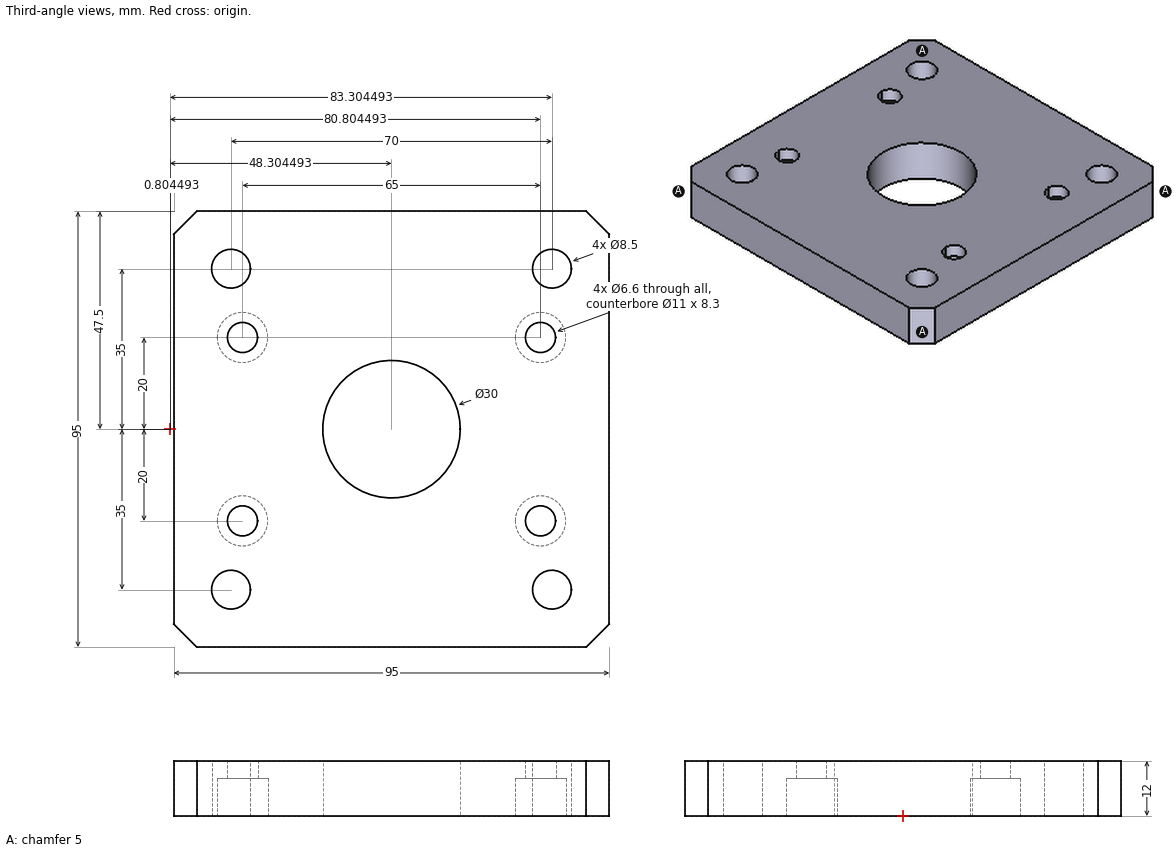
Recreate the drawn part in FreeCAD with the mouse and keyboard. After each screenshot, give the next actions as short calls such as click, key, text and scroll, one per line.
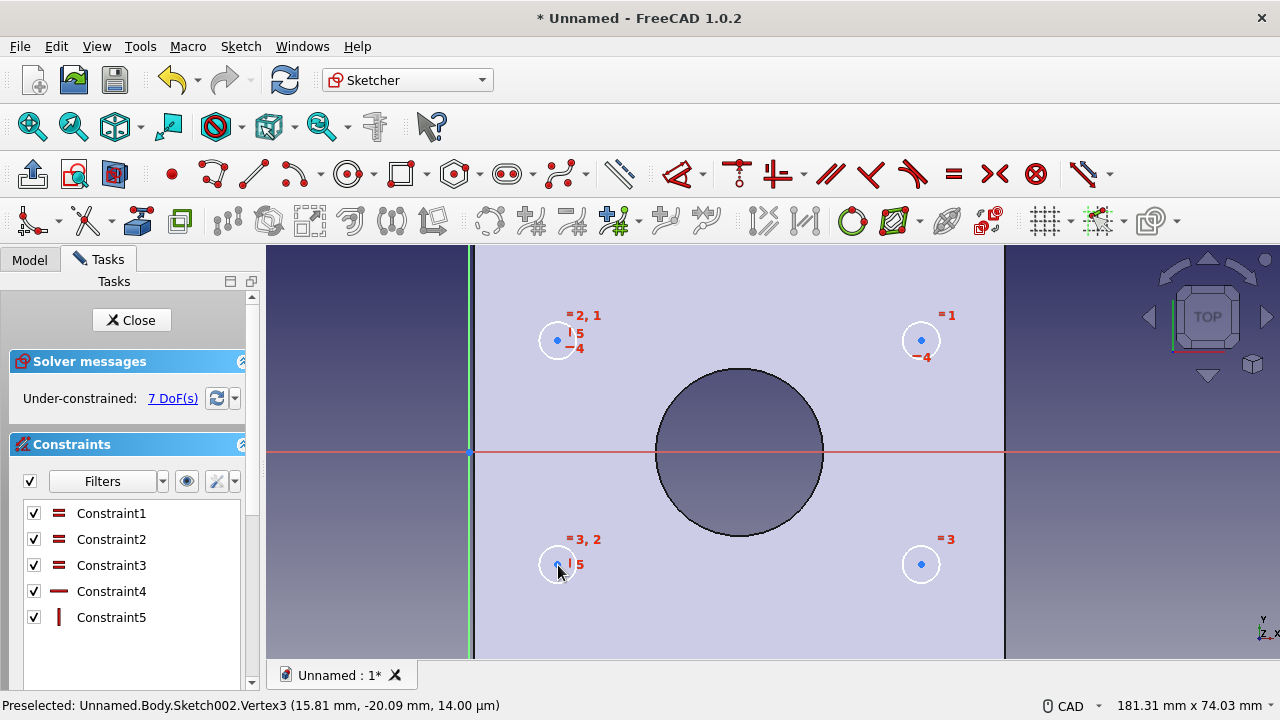
click(921, 341)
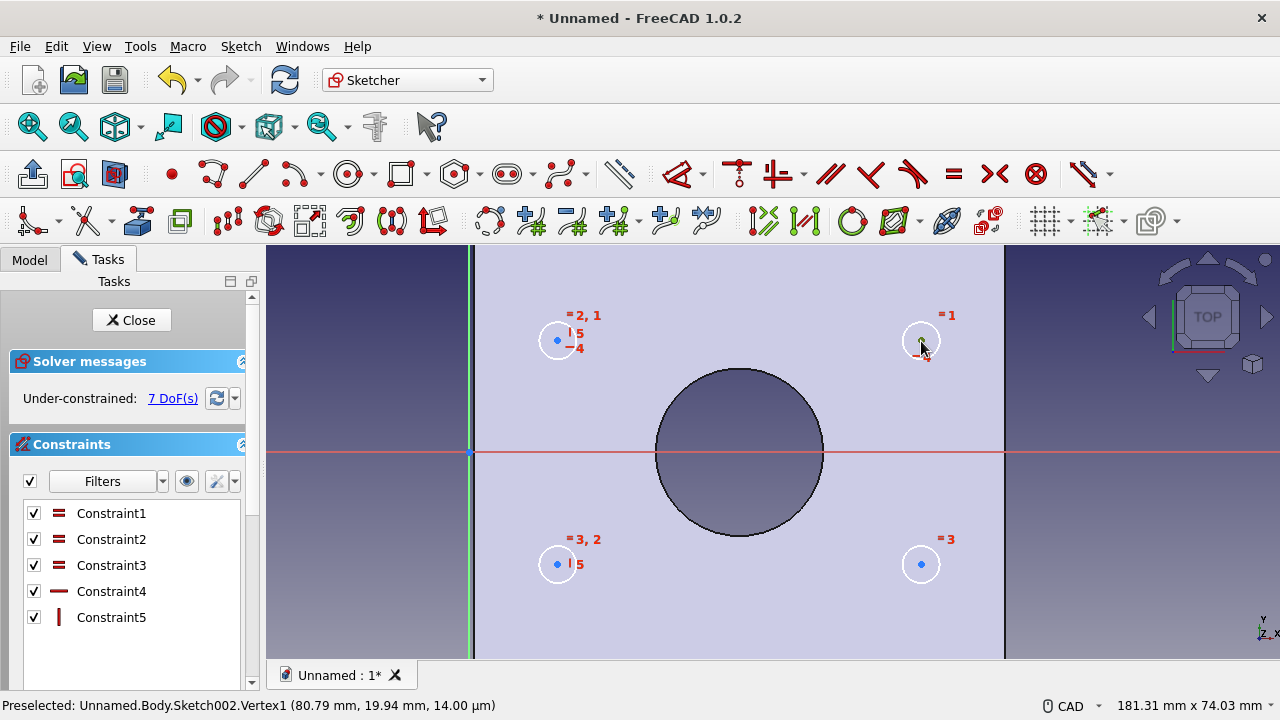
click(921, 565)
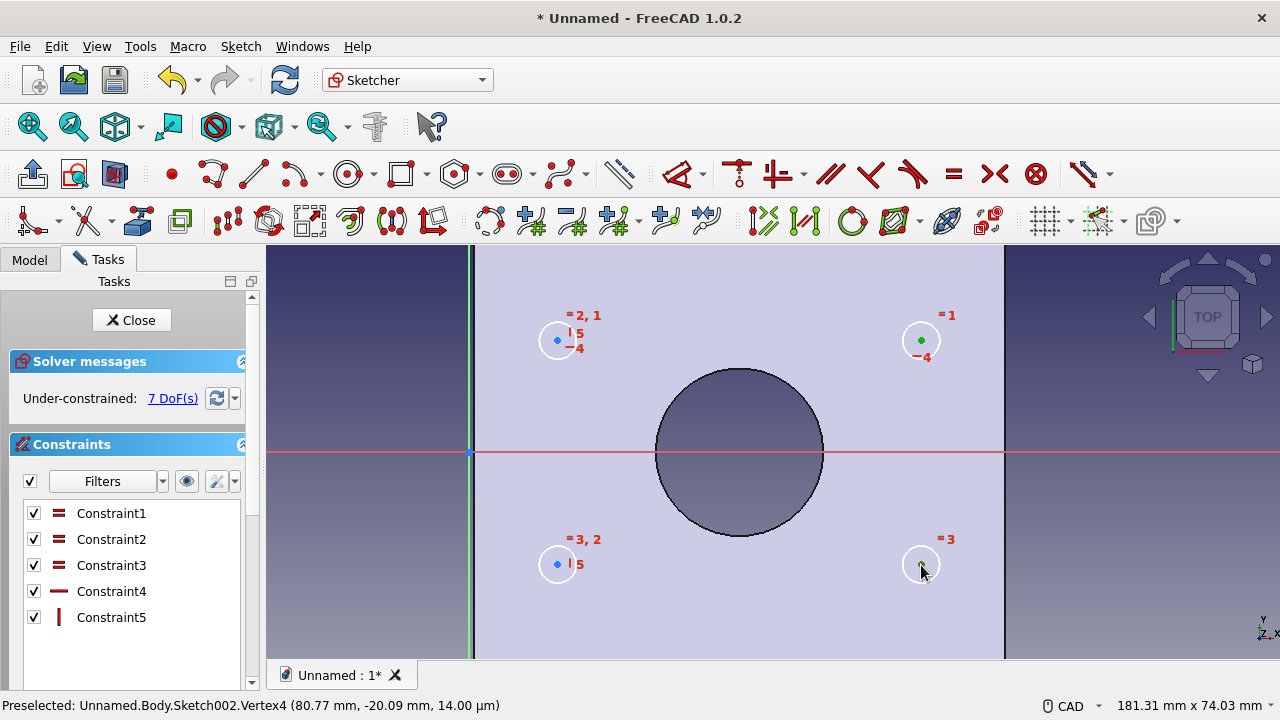
key(v)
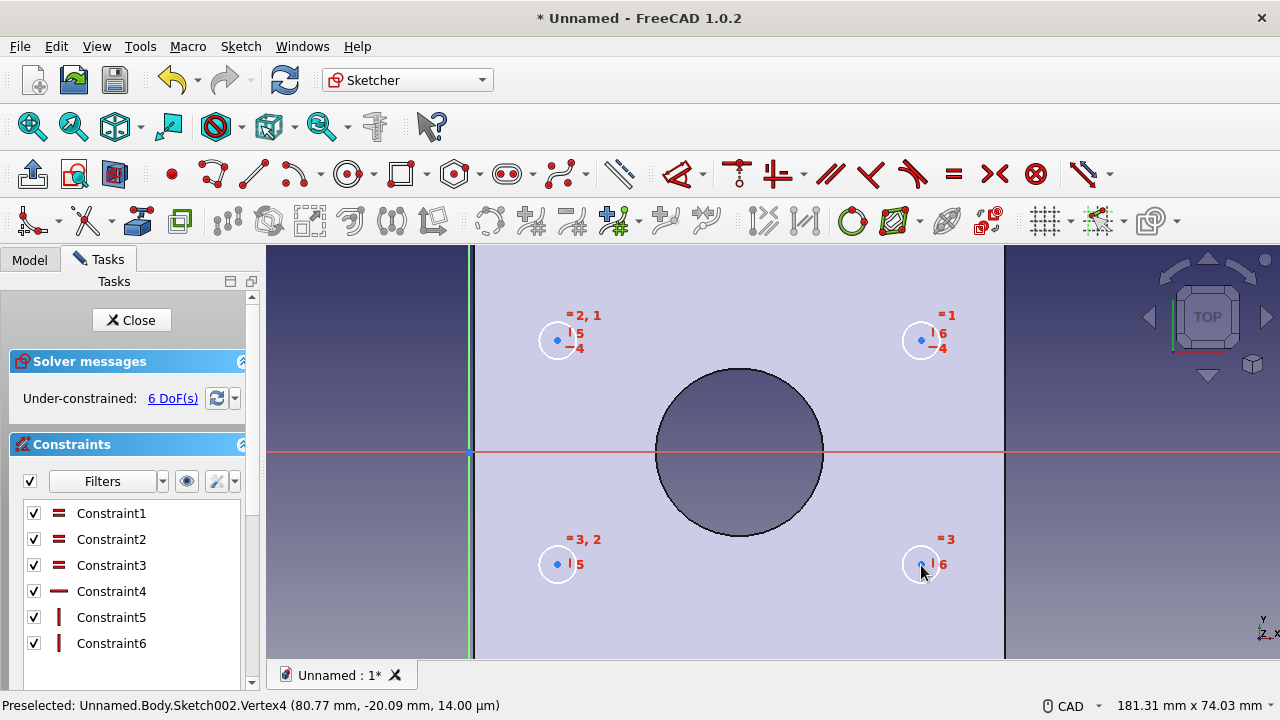
click(558, 565)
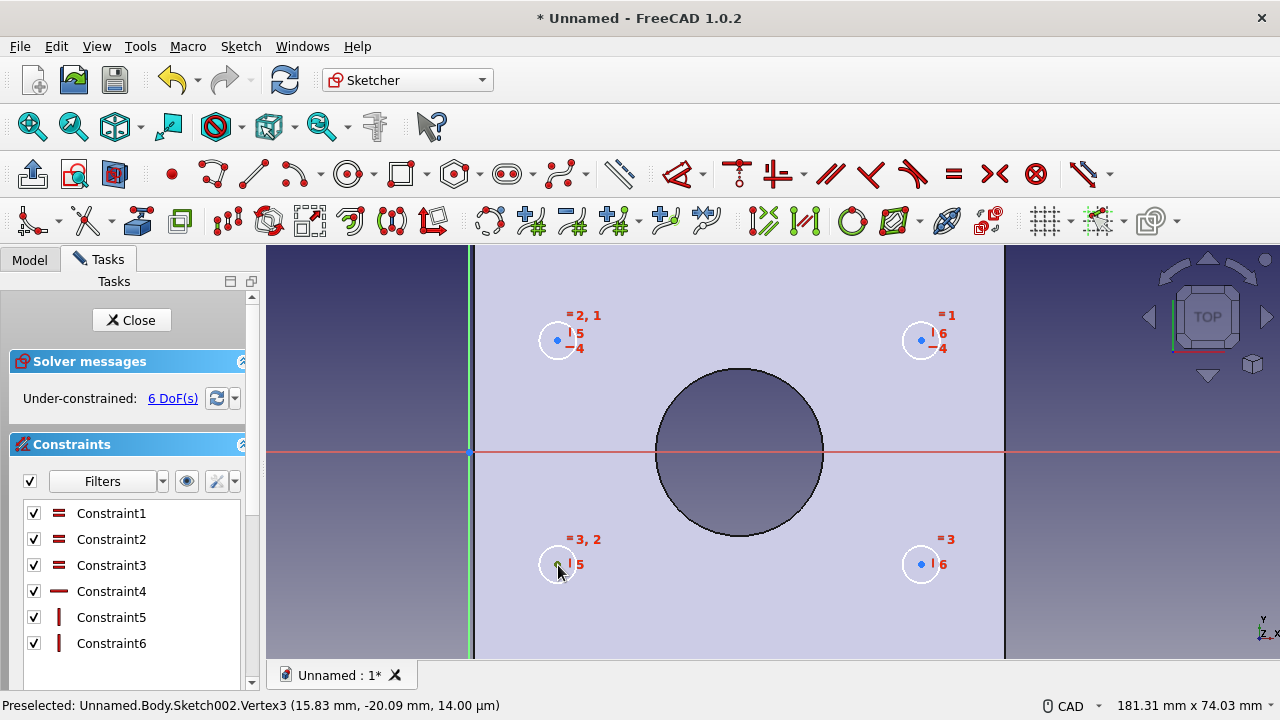
click(921, 565)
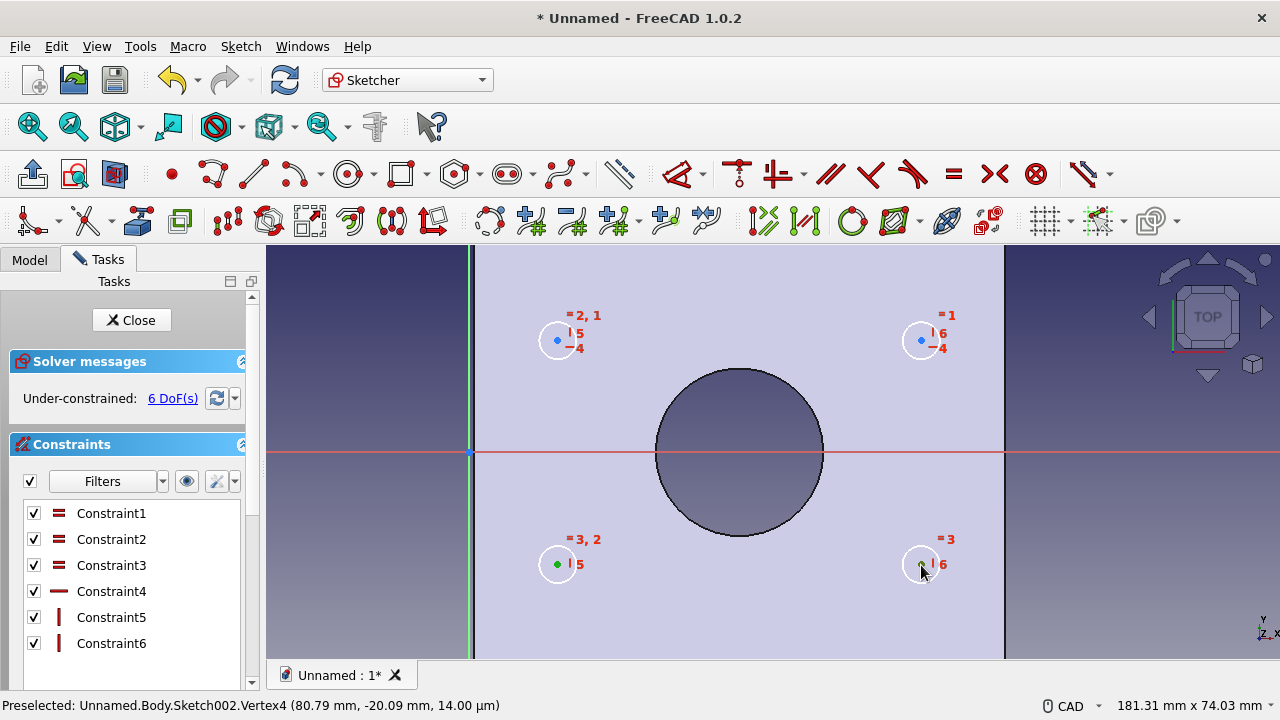
key(h)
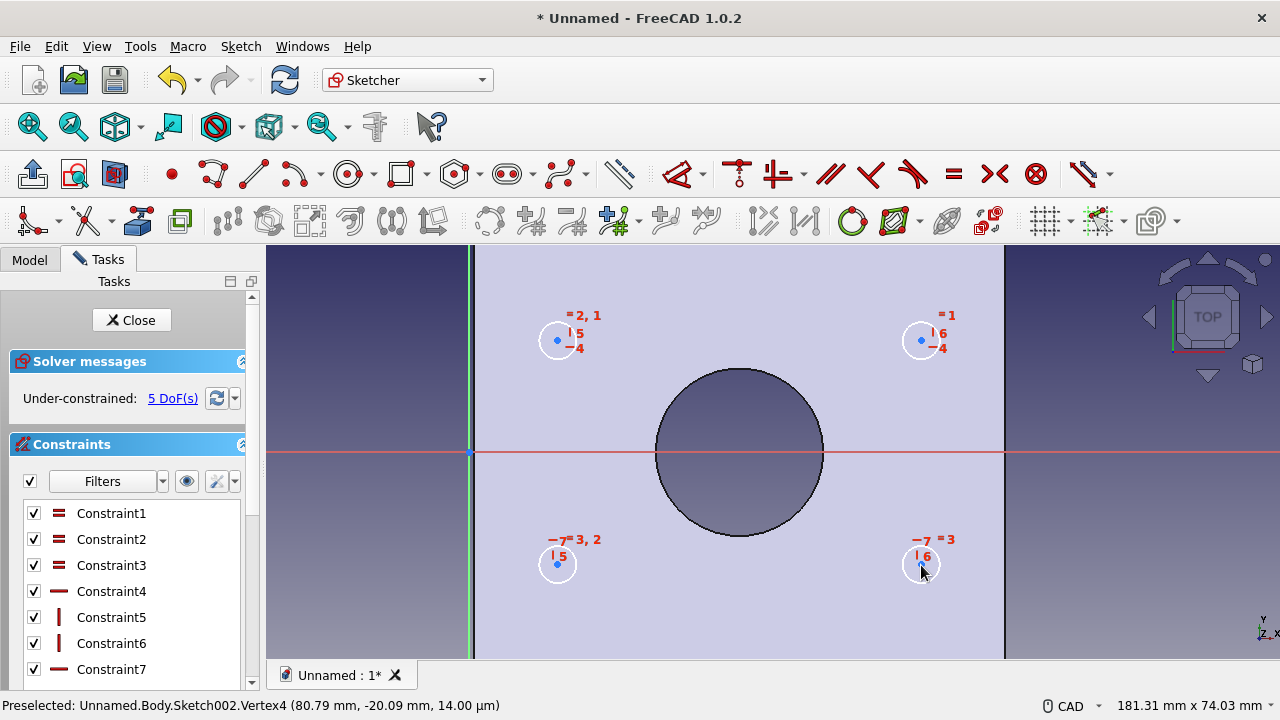
key(d)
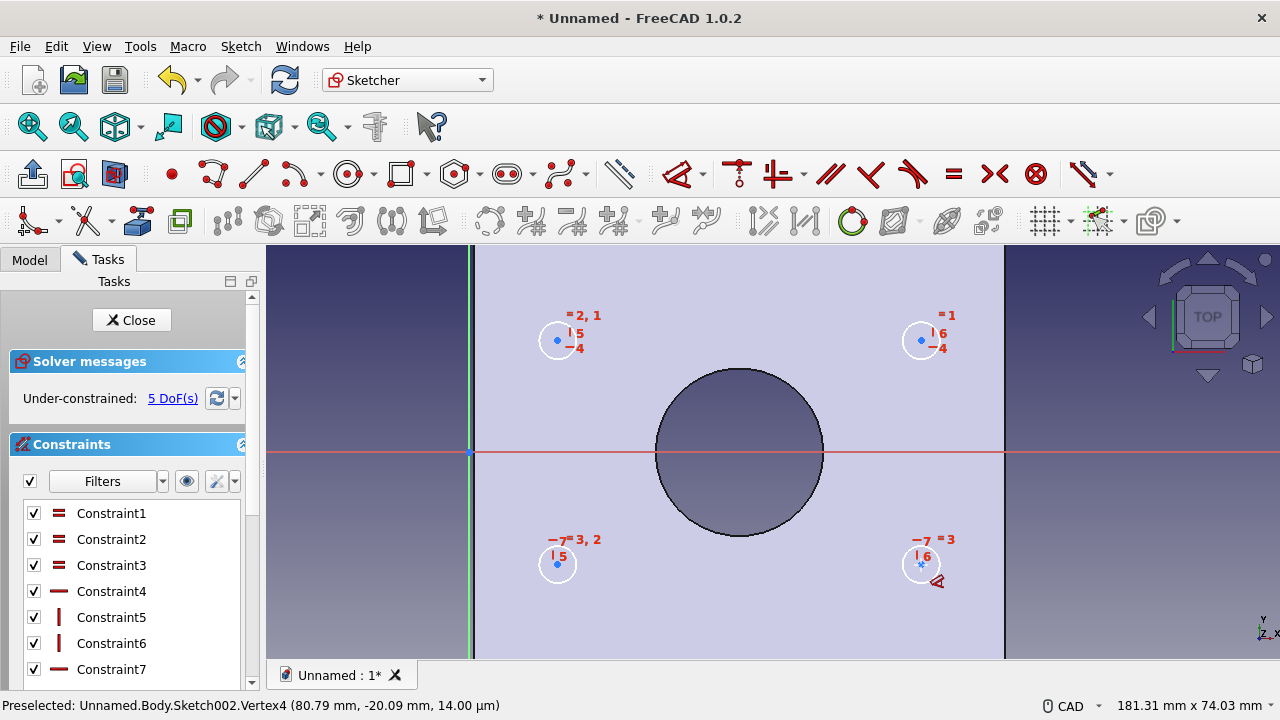
click(934, 328)
click(957, 305)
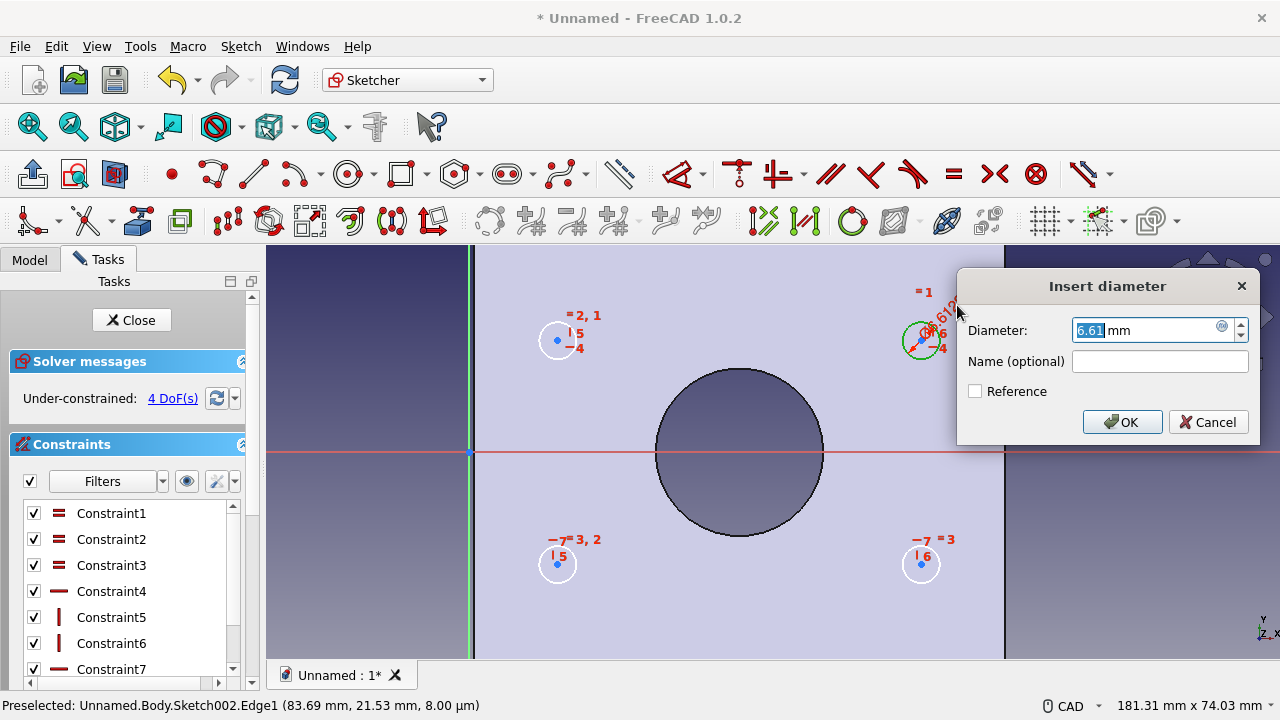
text(6.6)
key(Return)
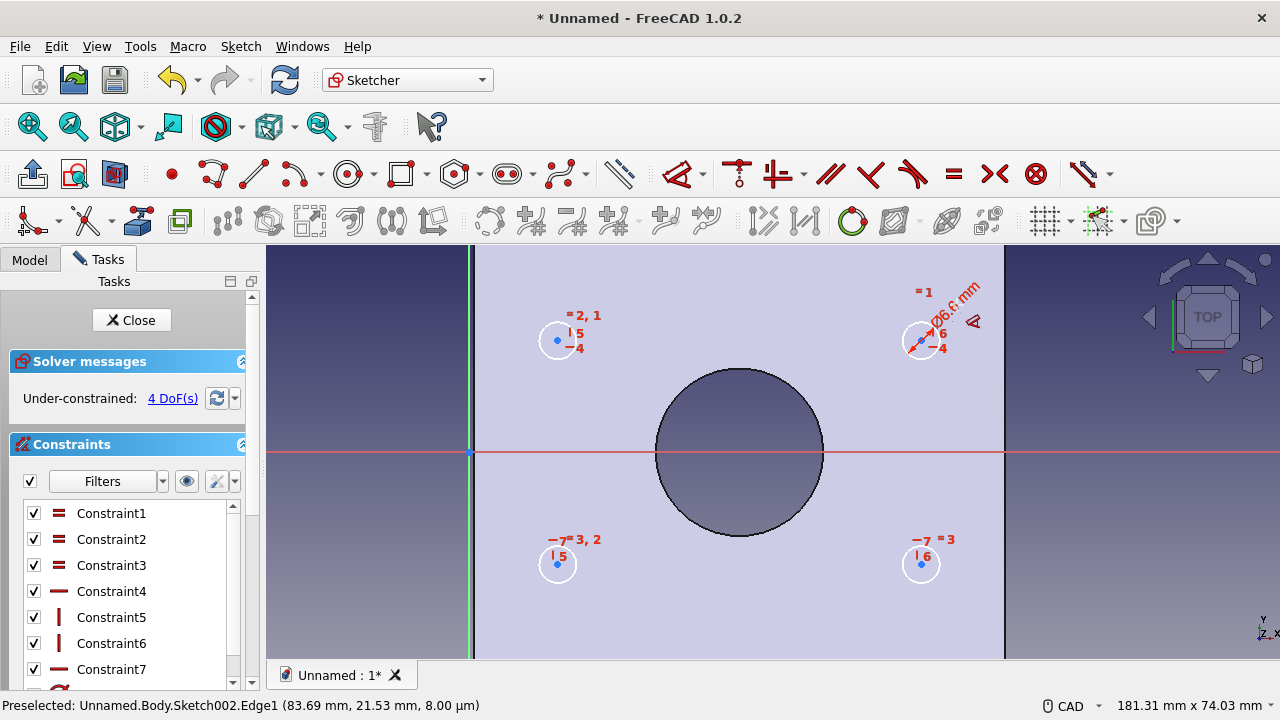
click(921, 341)
click(435, 396)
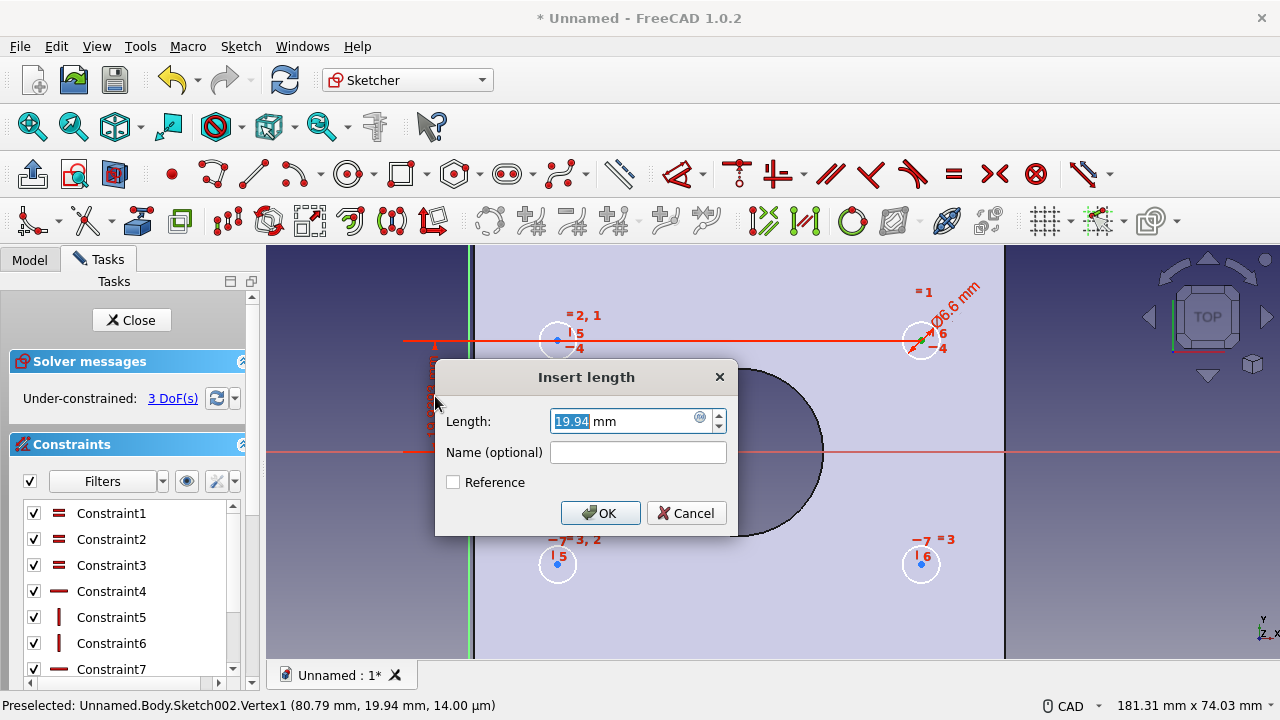
text(20)
key(Return)